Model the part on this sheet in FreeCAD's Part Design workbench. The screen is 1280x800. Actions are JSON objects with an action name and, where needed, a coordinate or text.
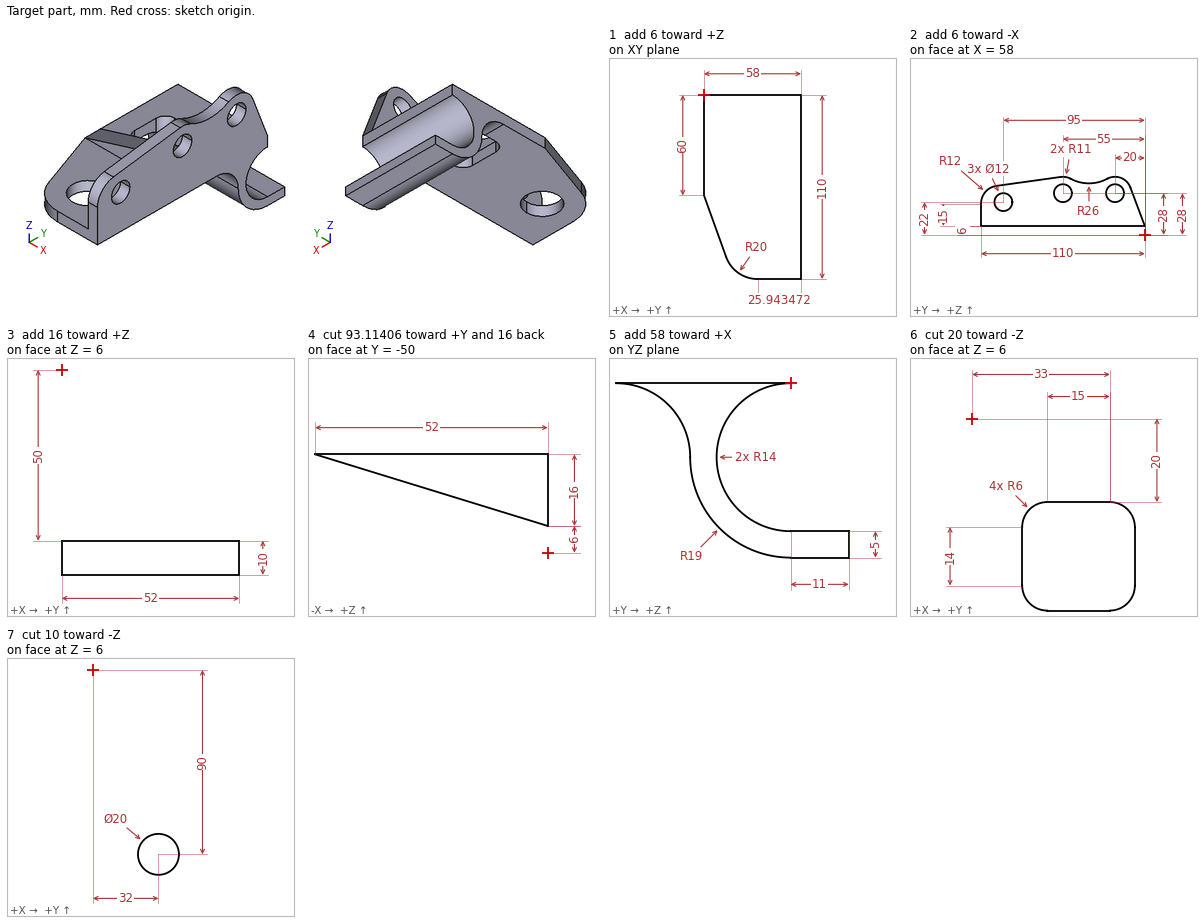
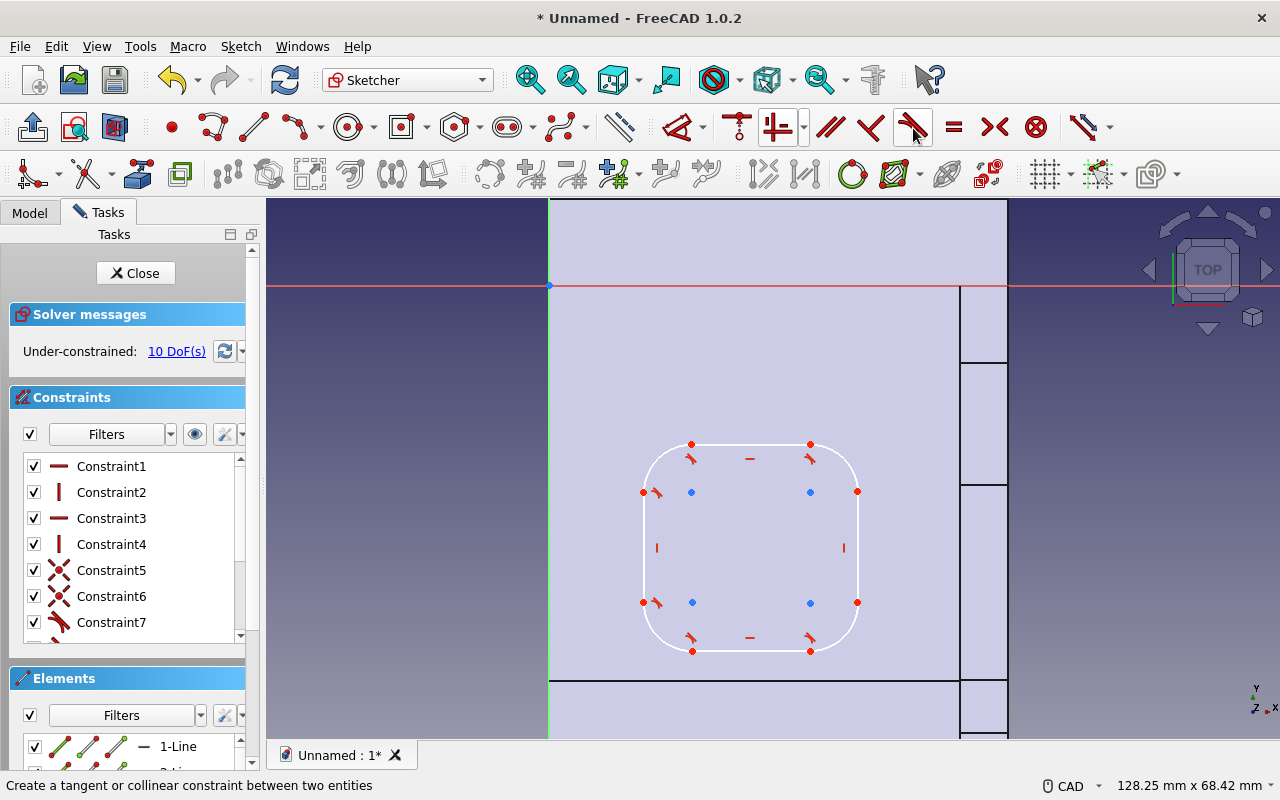
{"action": "left_click", "coordinate": [858, 570]}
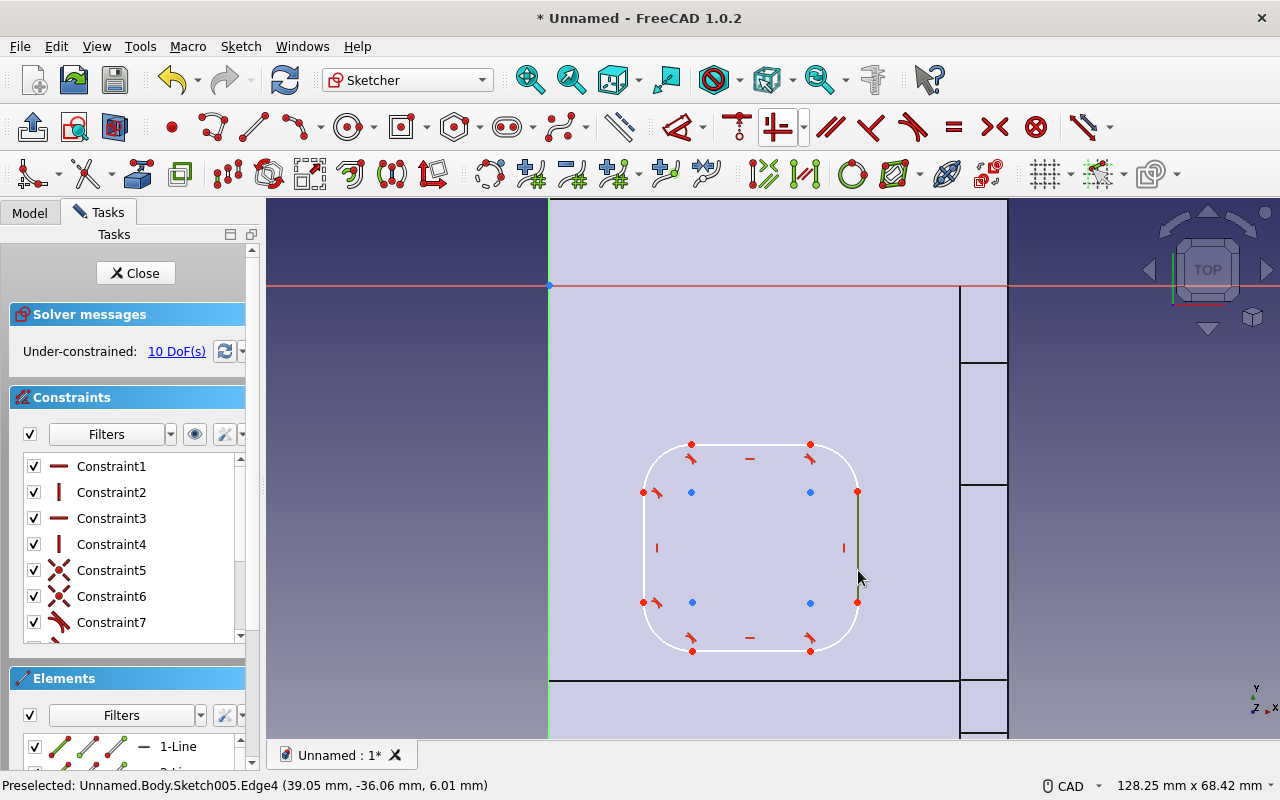
{"action": "left_click", "coordinate": [832, 646]}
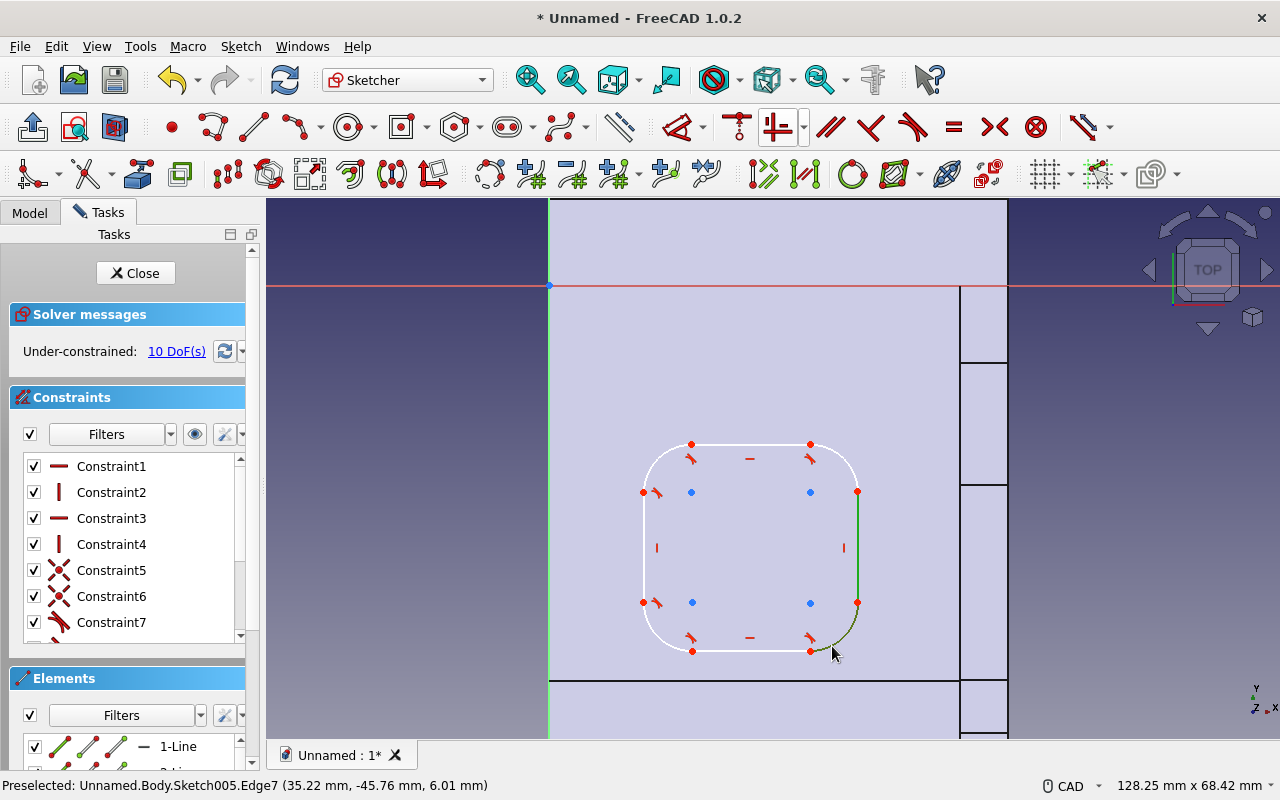
{"action": "left_click", "coordinate": [913, 128]}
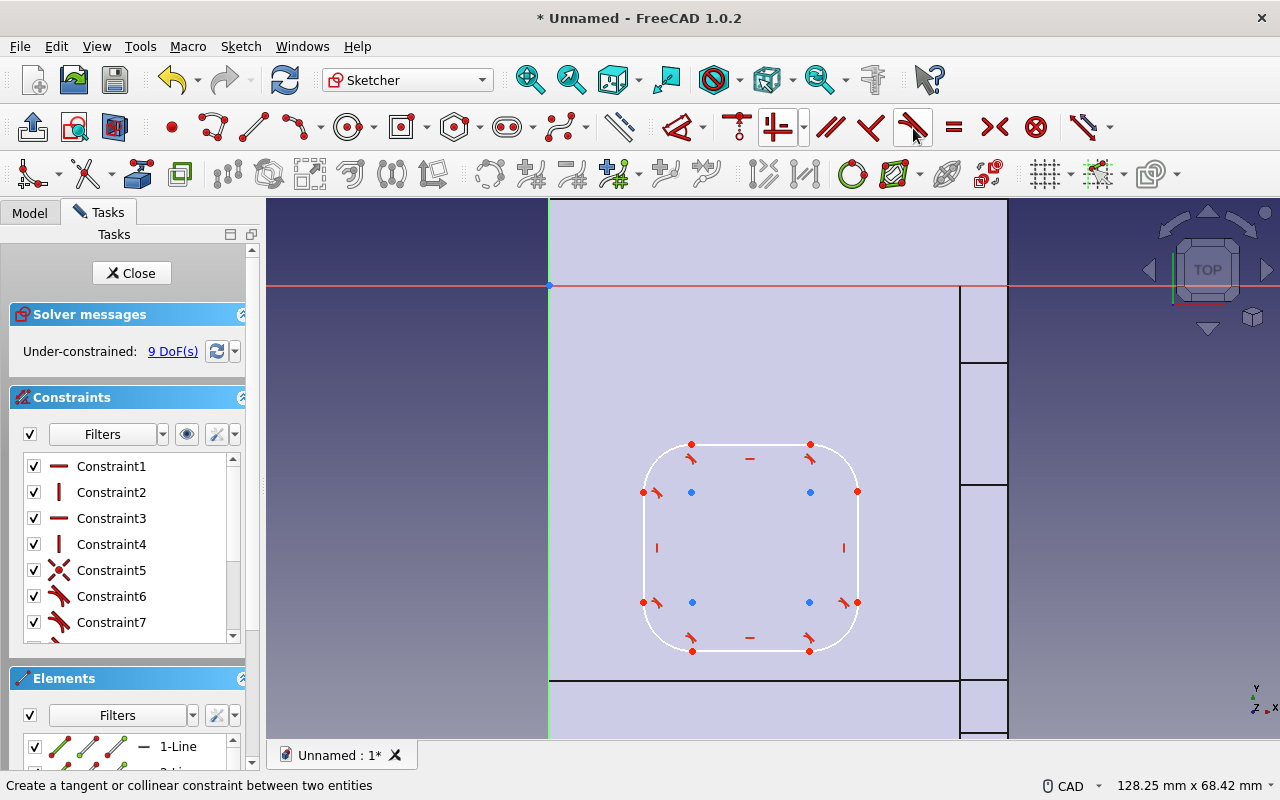
{"action": "left_click", "coordinate": [858, 570]}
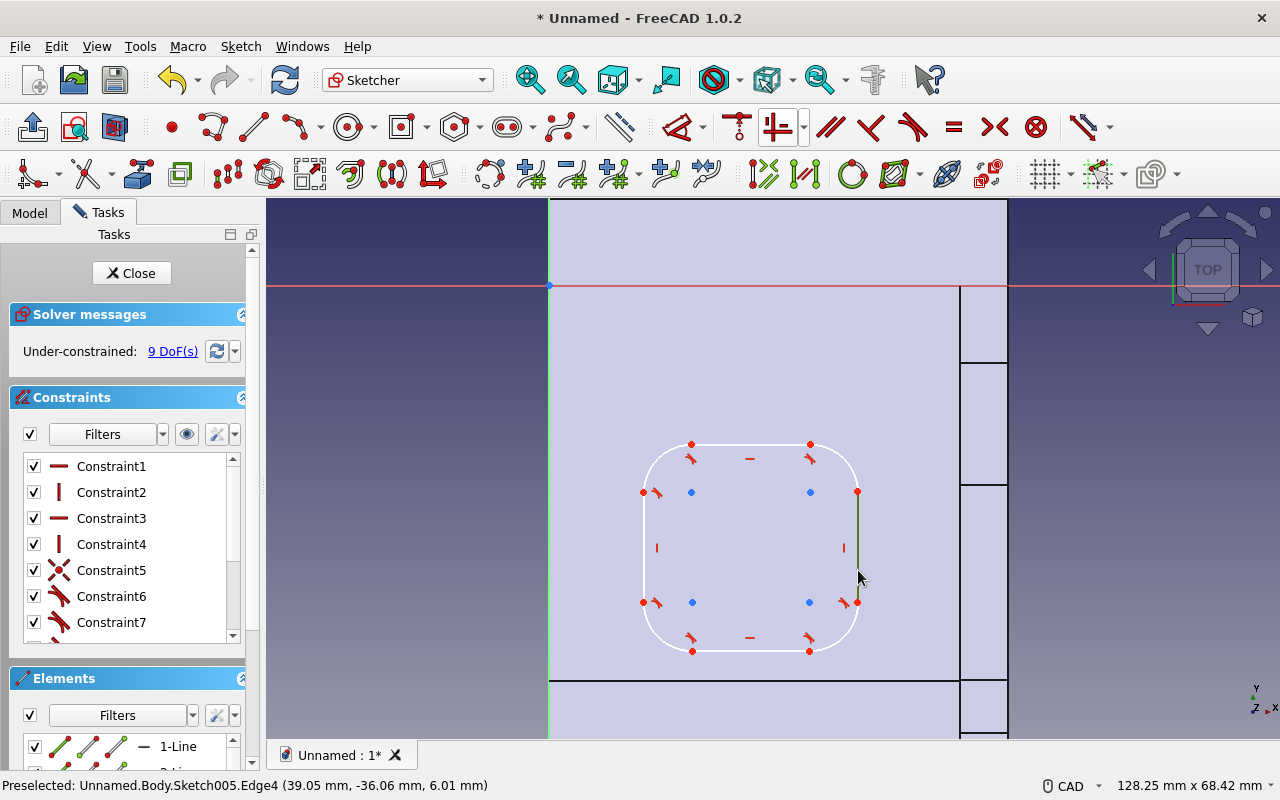
{"action": "left_click", "coordinate": [853, 471]}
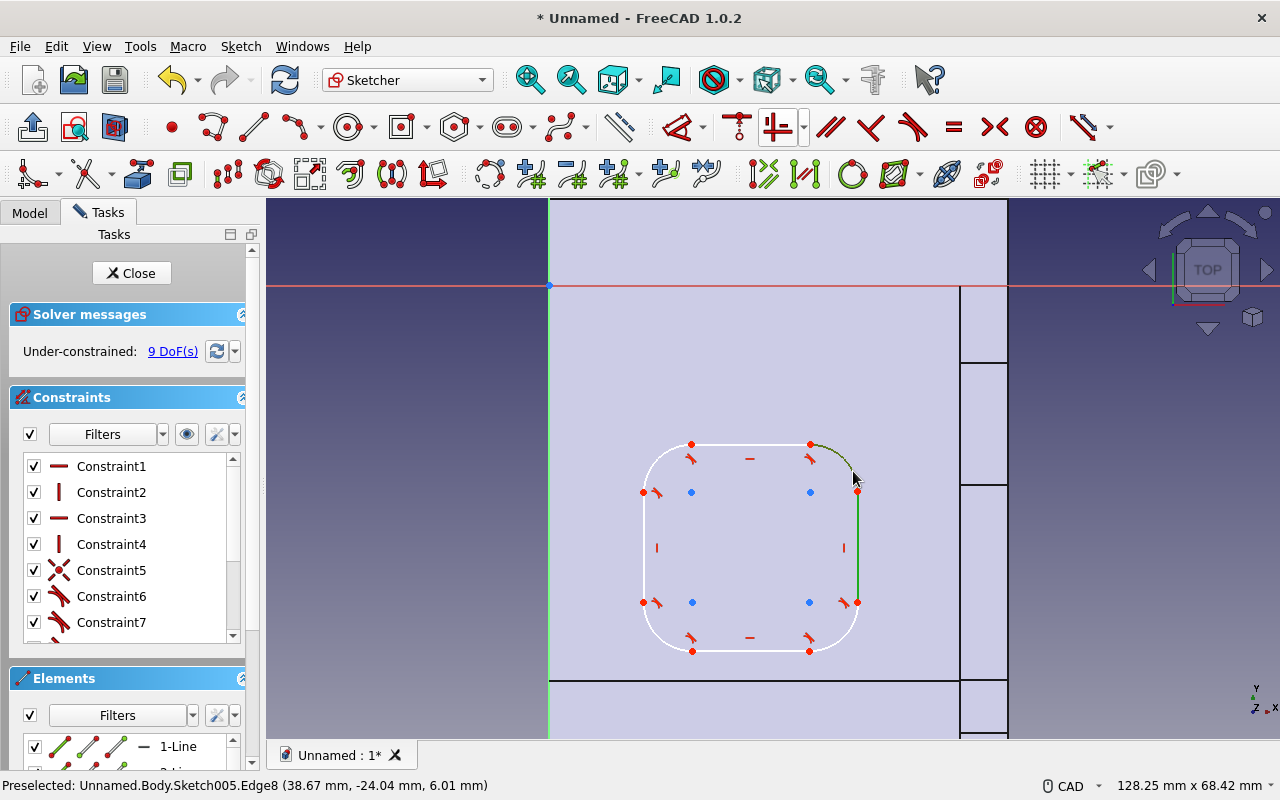
{"action": "left_click", "coordinate": [913, 128]}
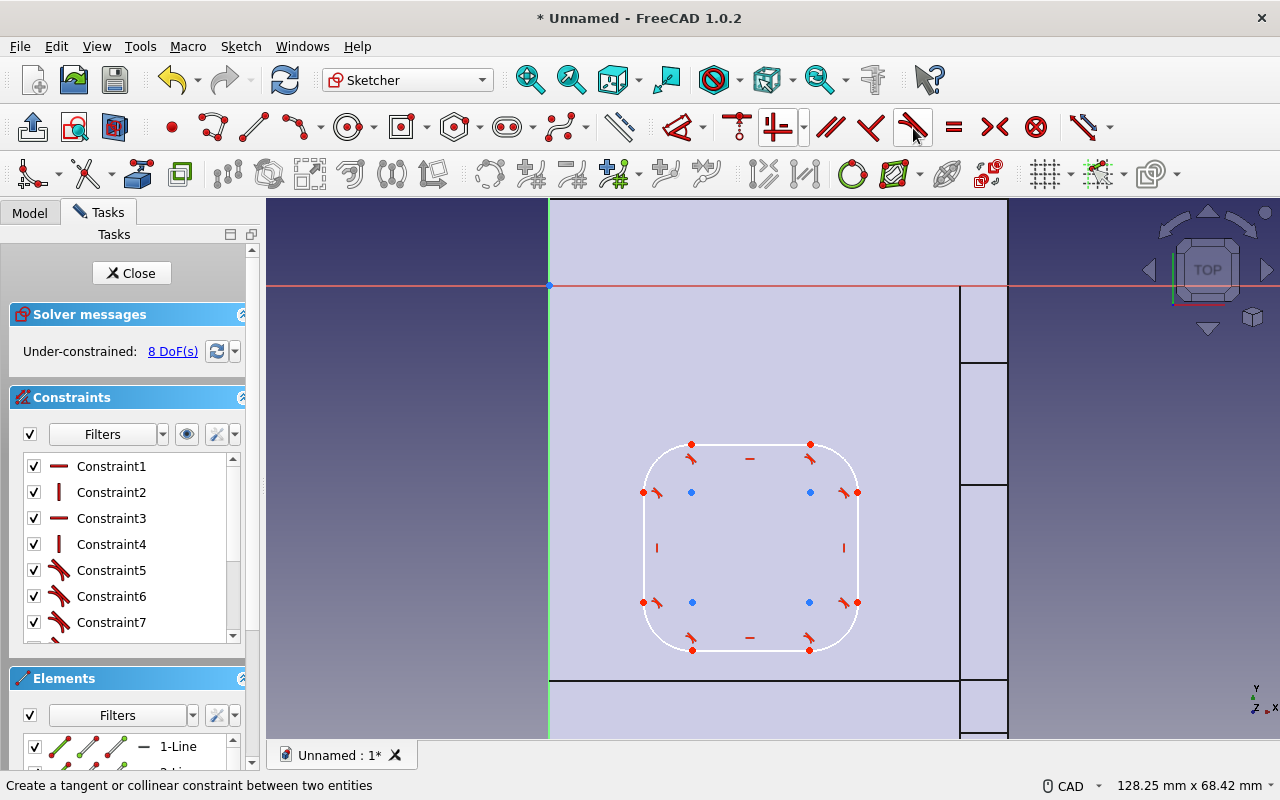
{"action": "left_click", "coordinate": [670, 450]}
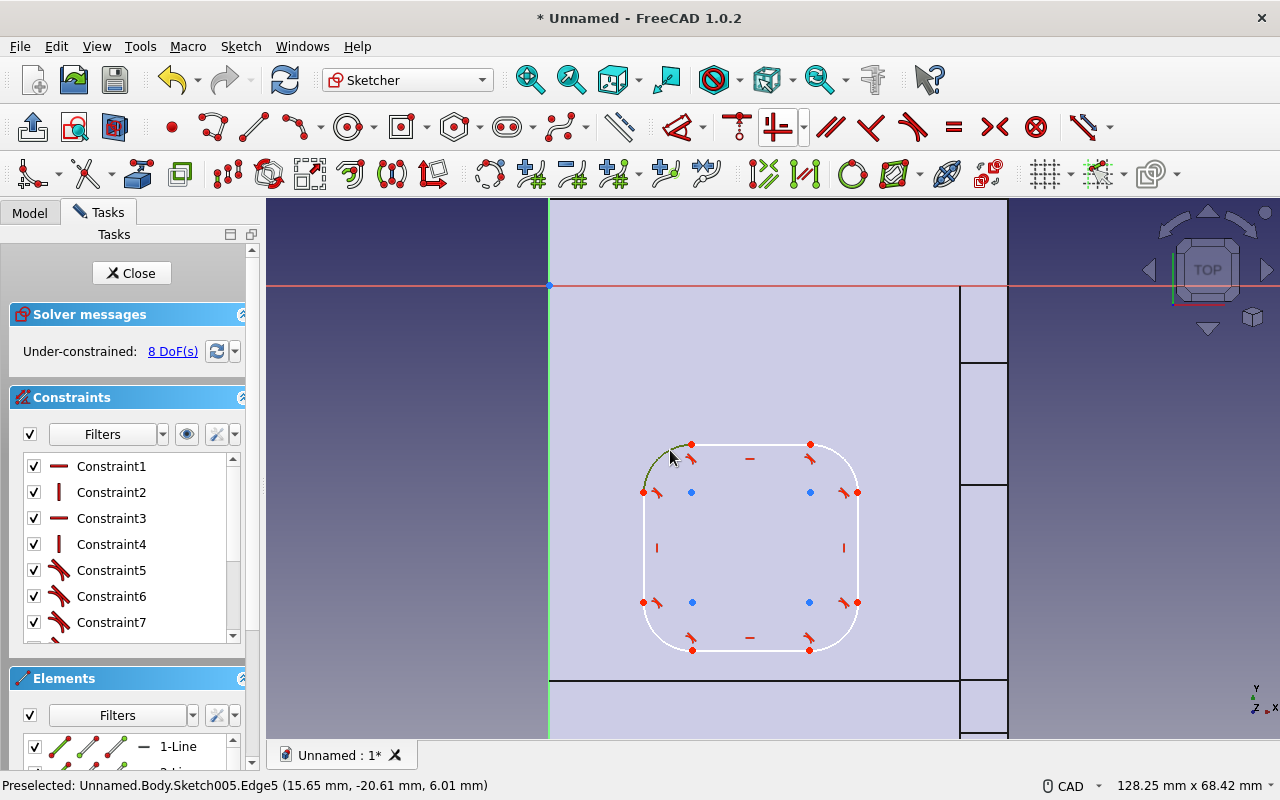
{"action": "left_click", "coordinate": [649, 625]}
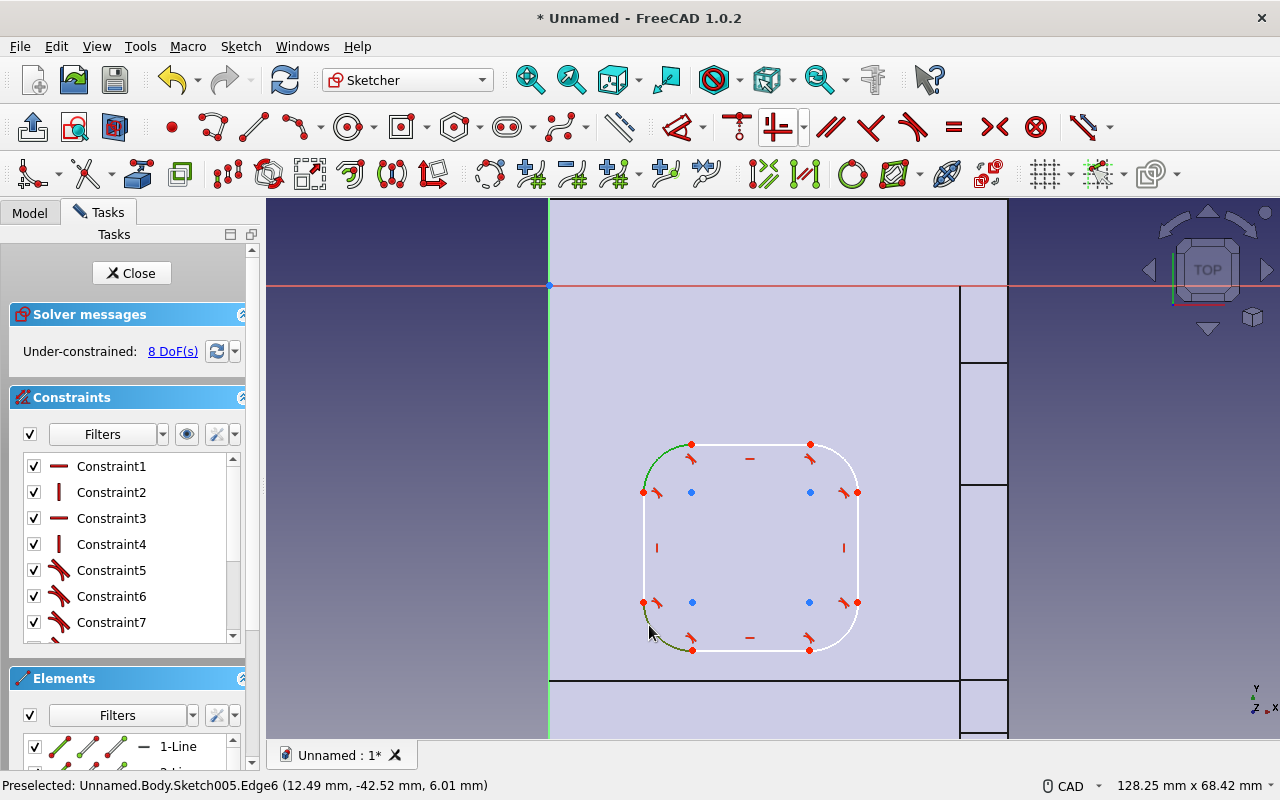
{"action": "left_click", "coordinate": [832, 646]}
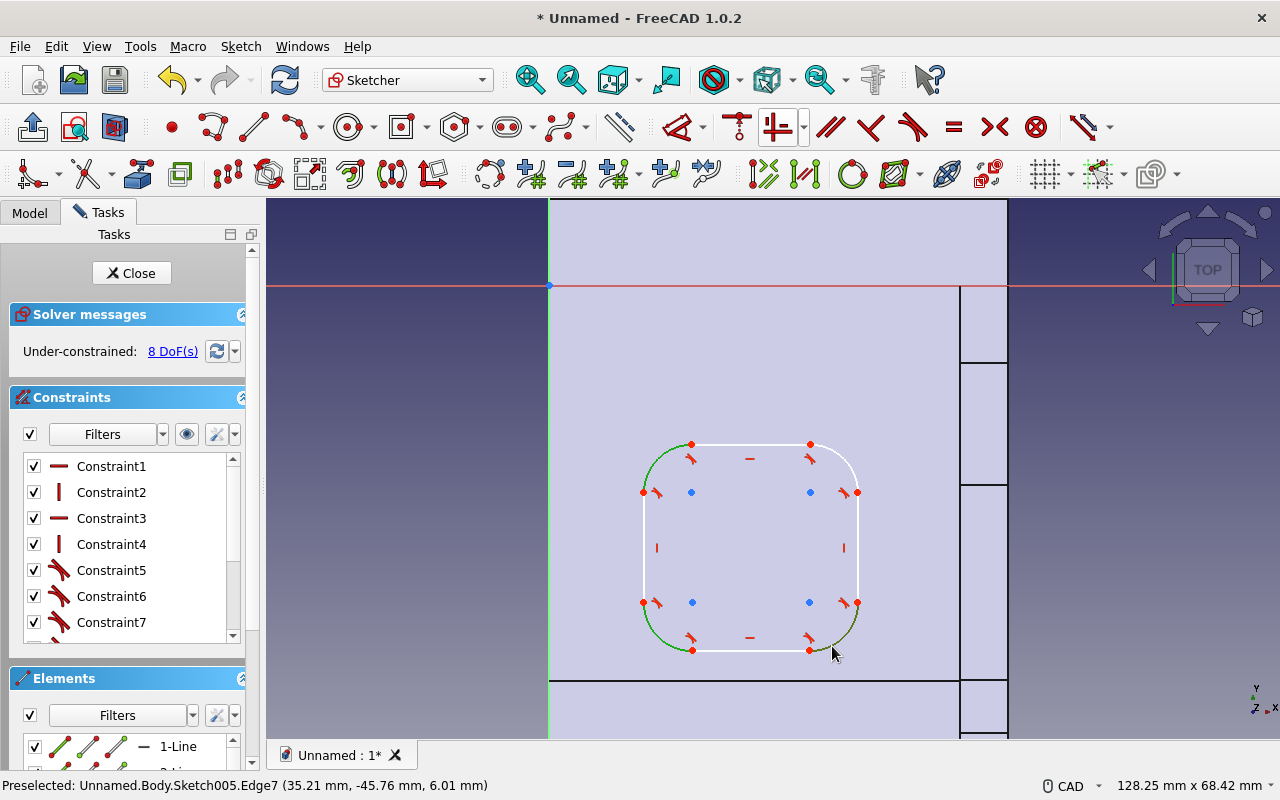
{"action": "left_click", "coordinate": [853, 471]}